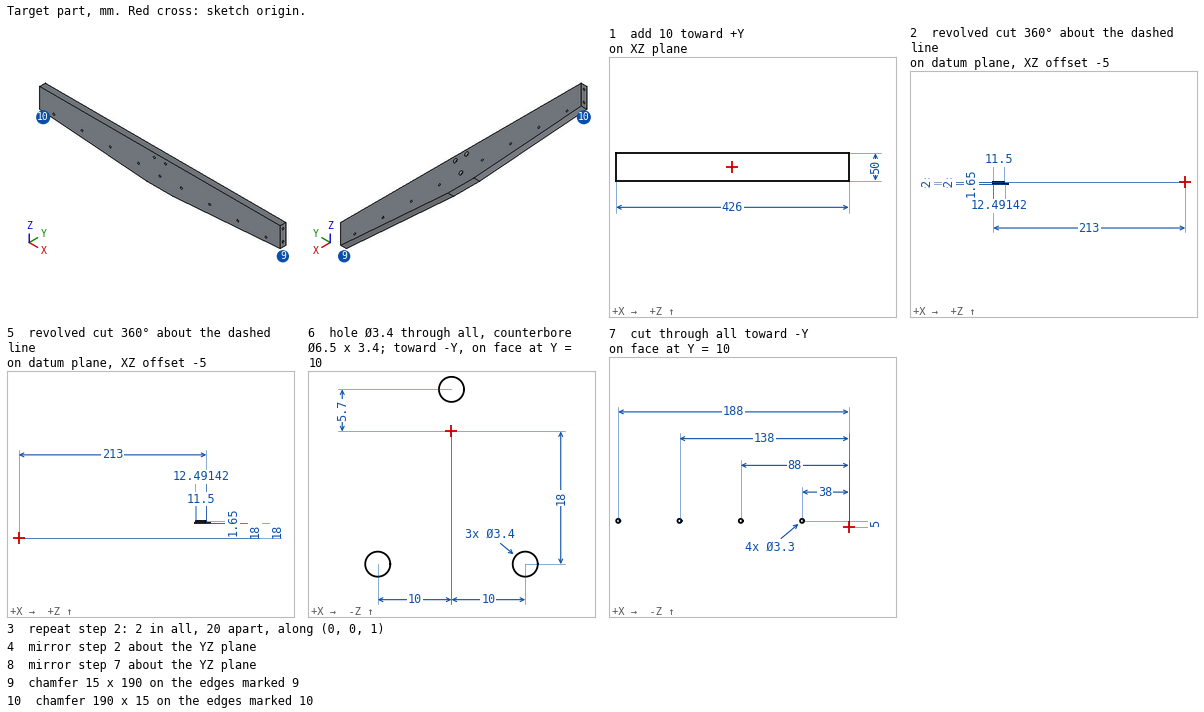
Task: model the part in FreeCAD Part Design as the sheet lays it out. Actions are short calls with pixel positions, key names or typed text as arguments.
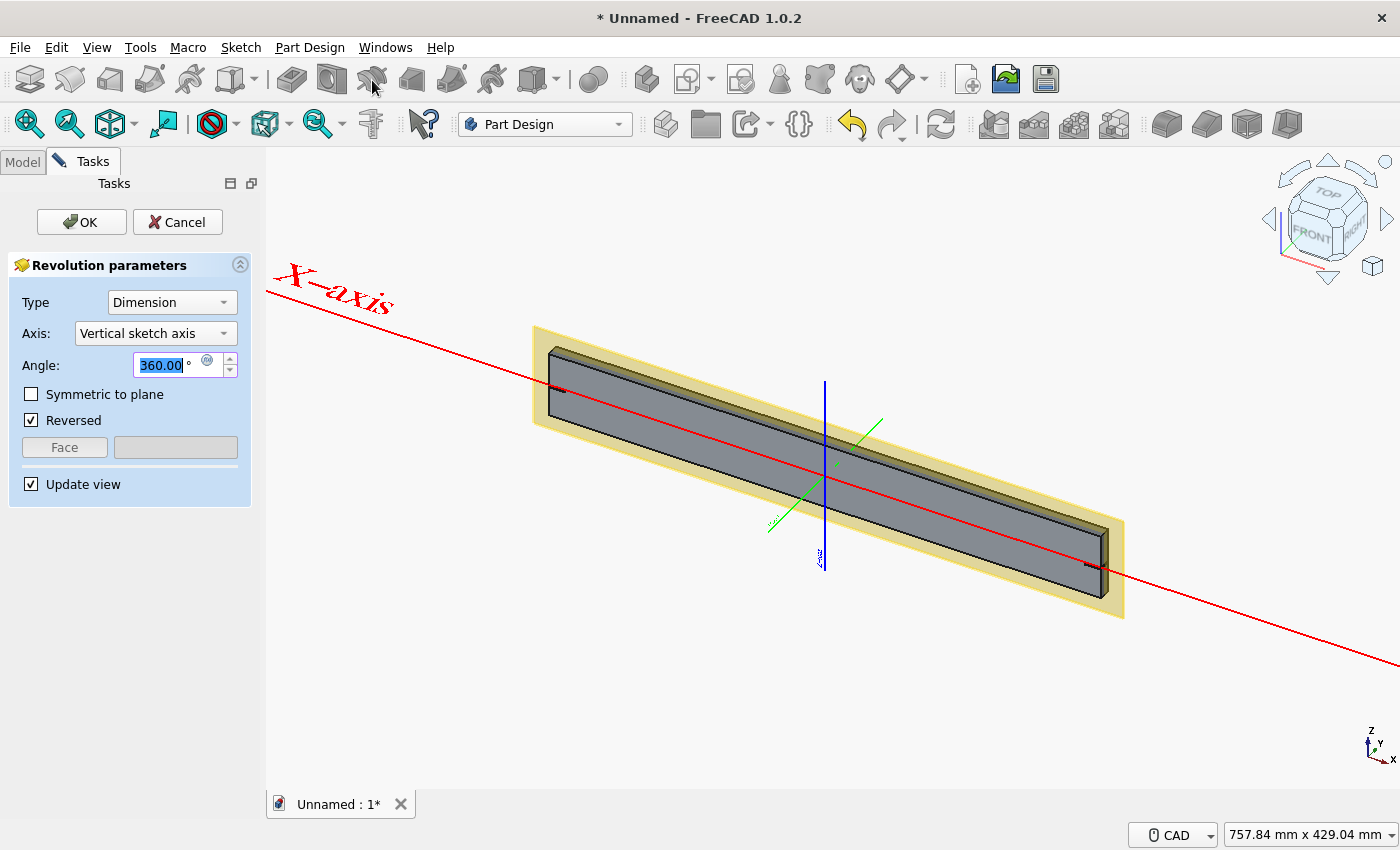
click(156, 334)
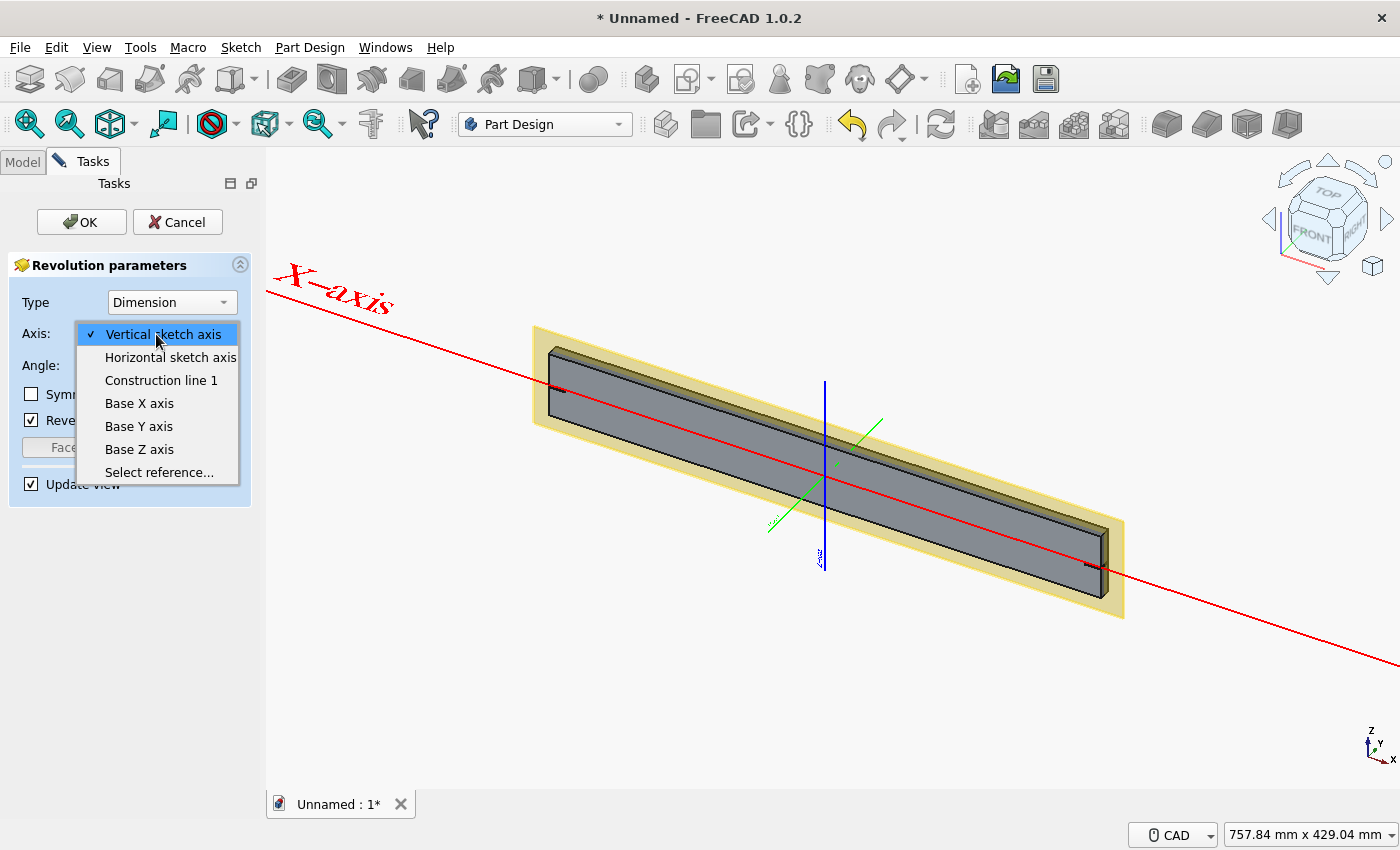
click(156, 380)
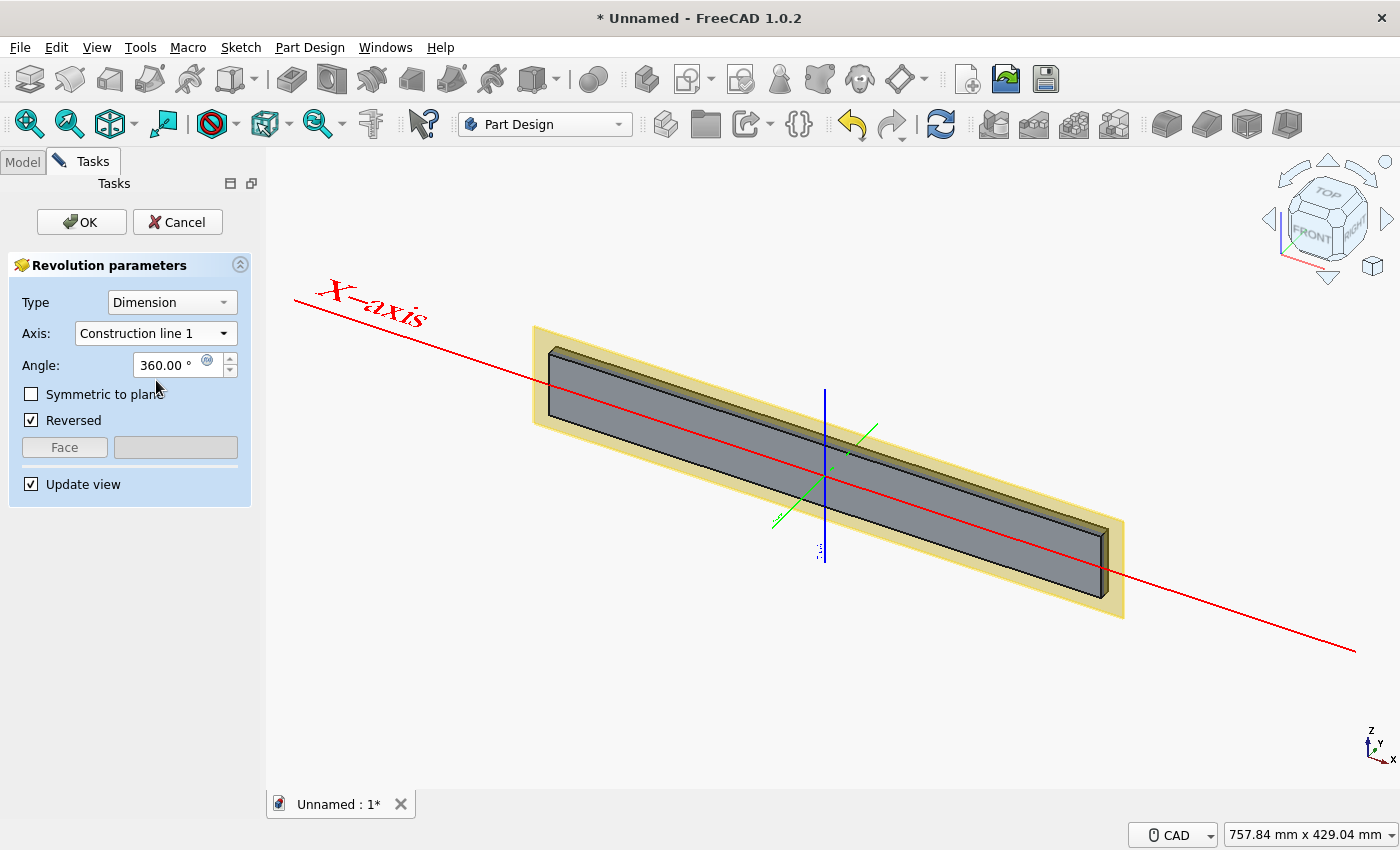
click(82, 222)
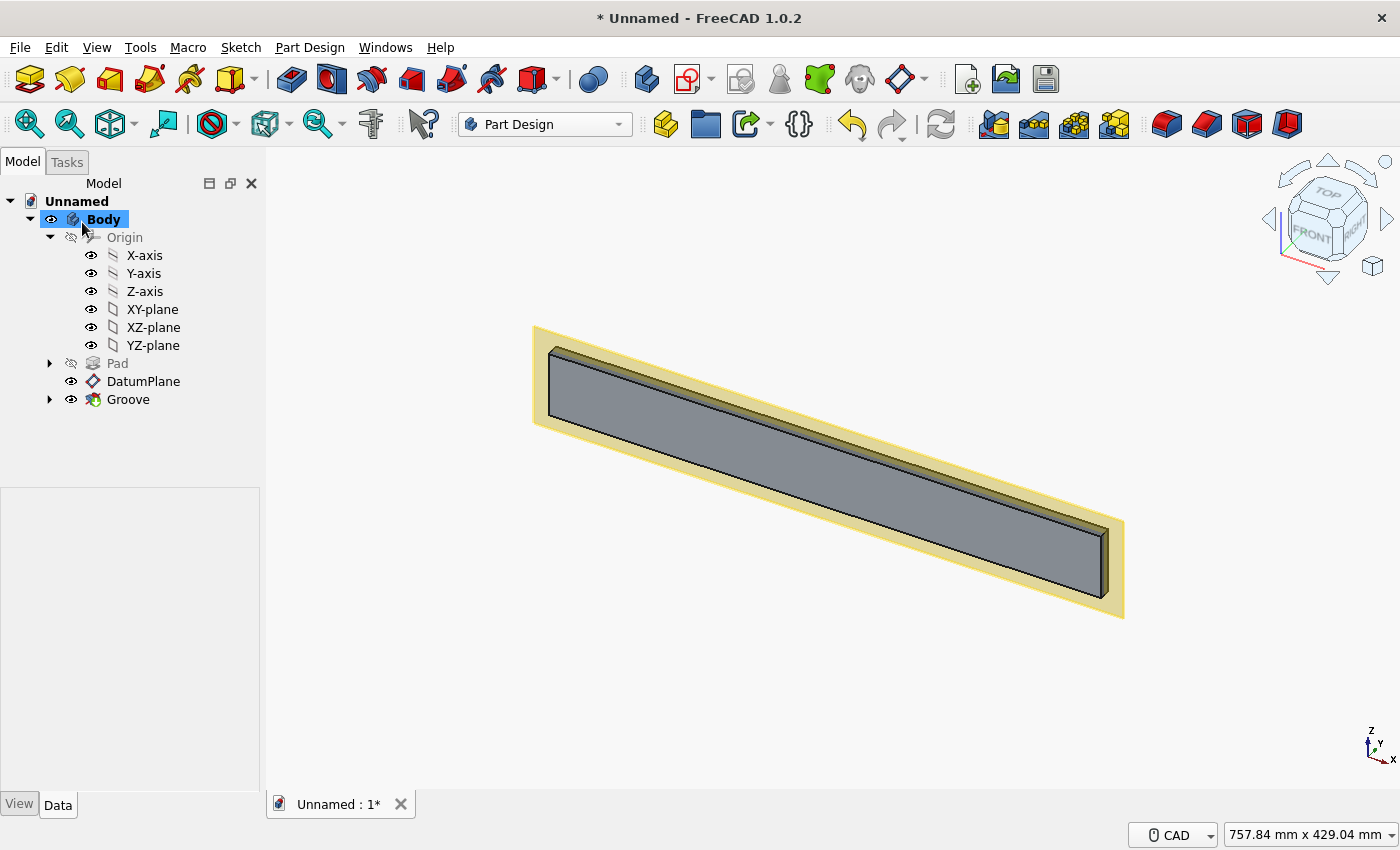
click(116, 381)
key(space)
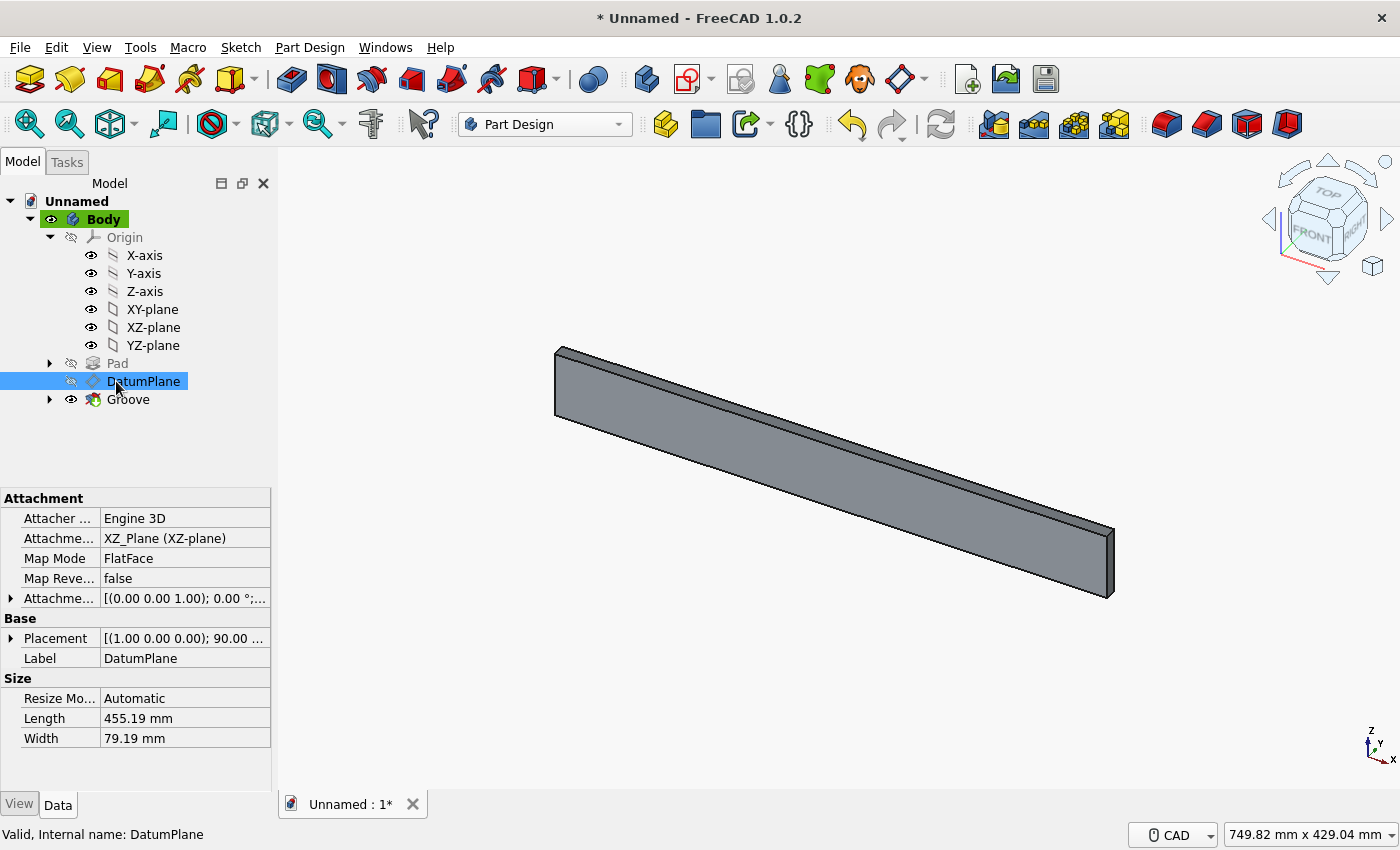
click(116, 399)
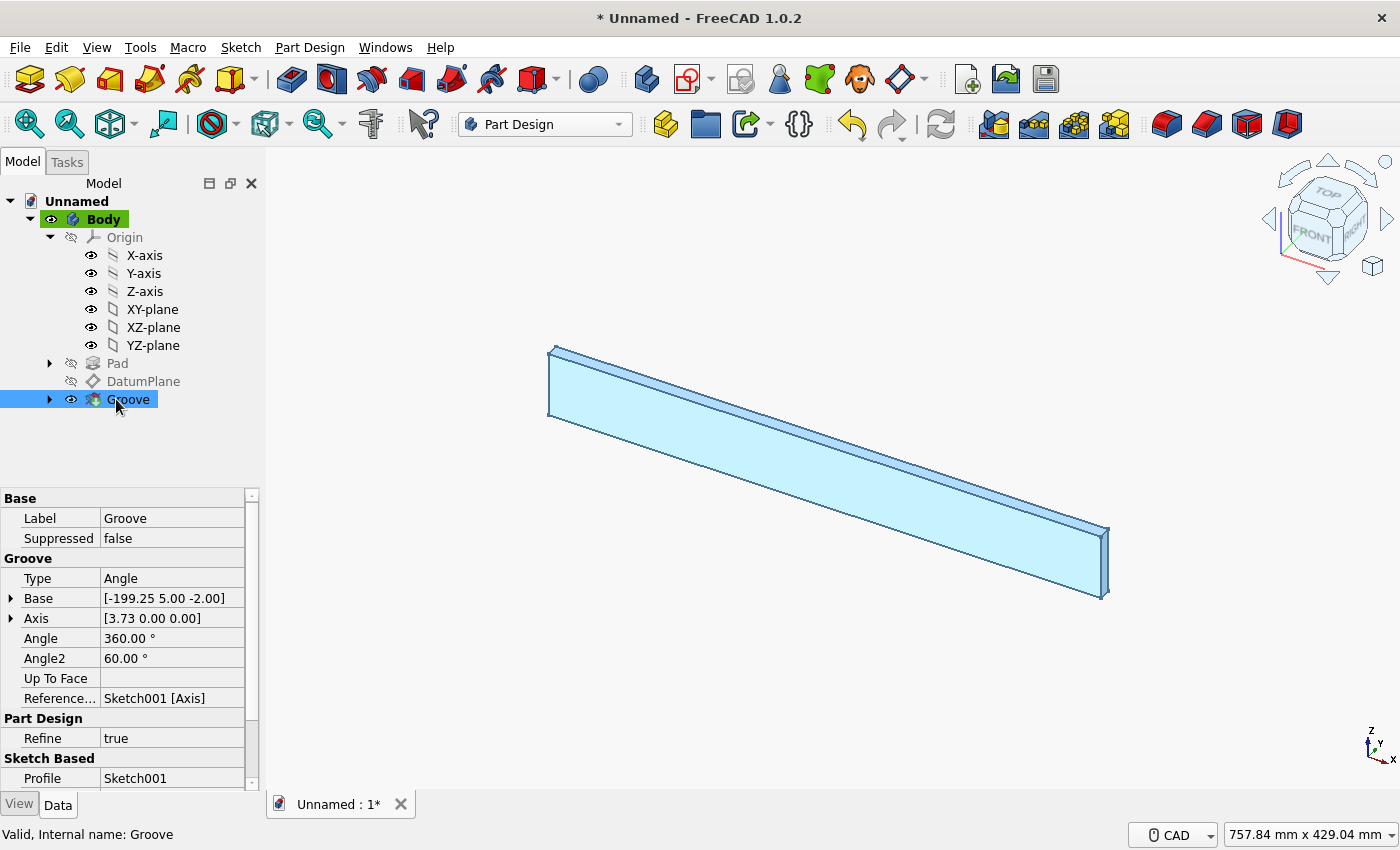
click(1034, 124)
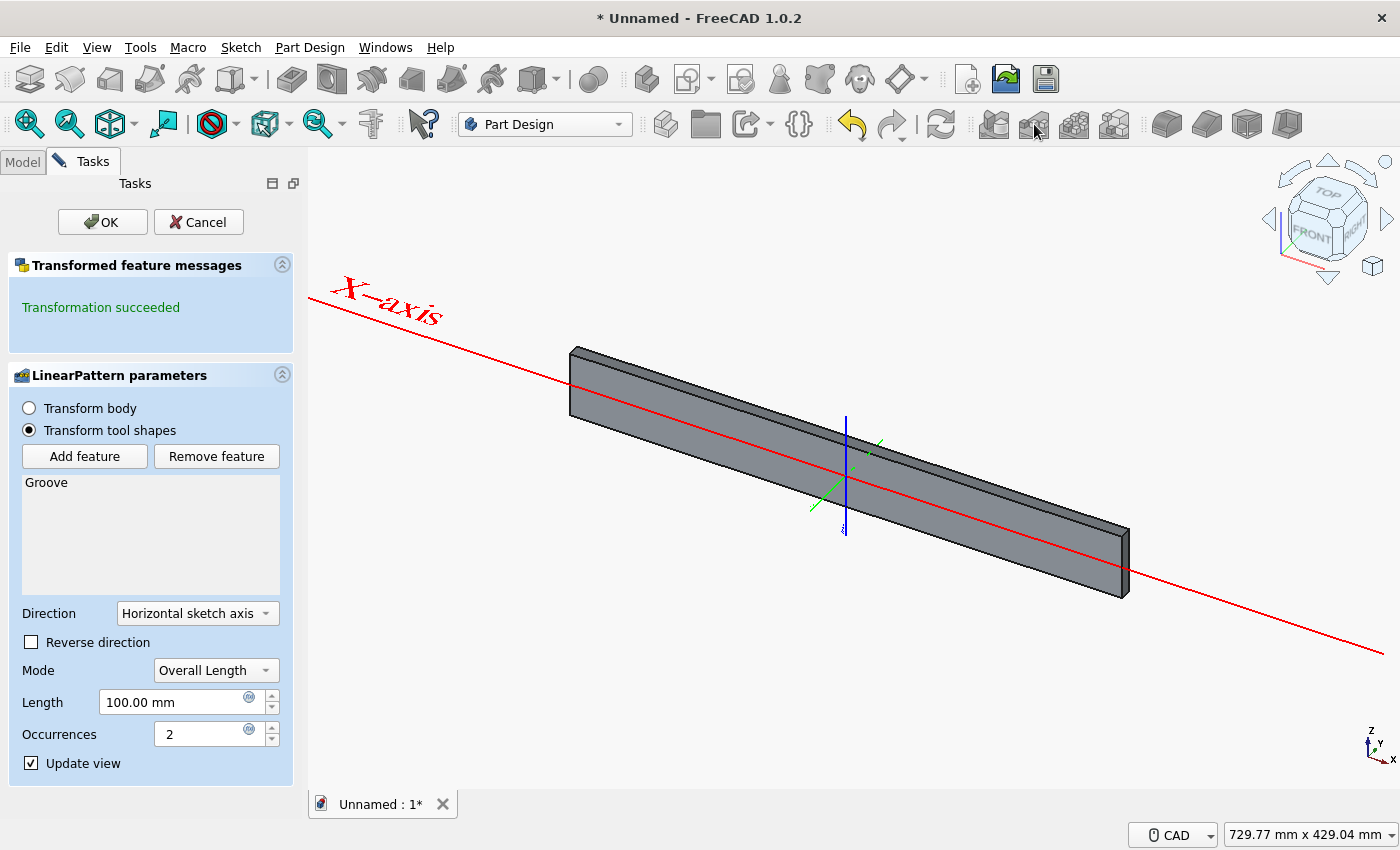
click(198, 614)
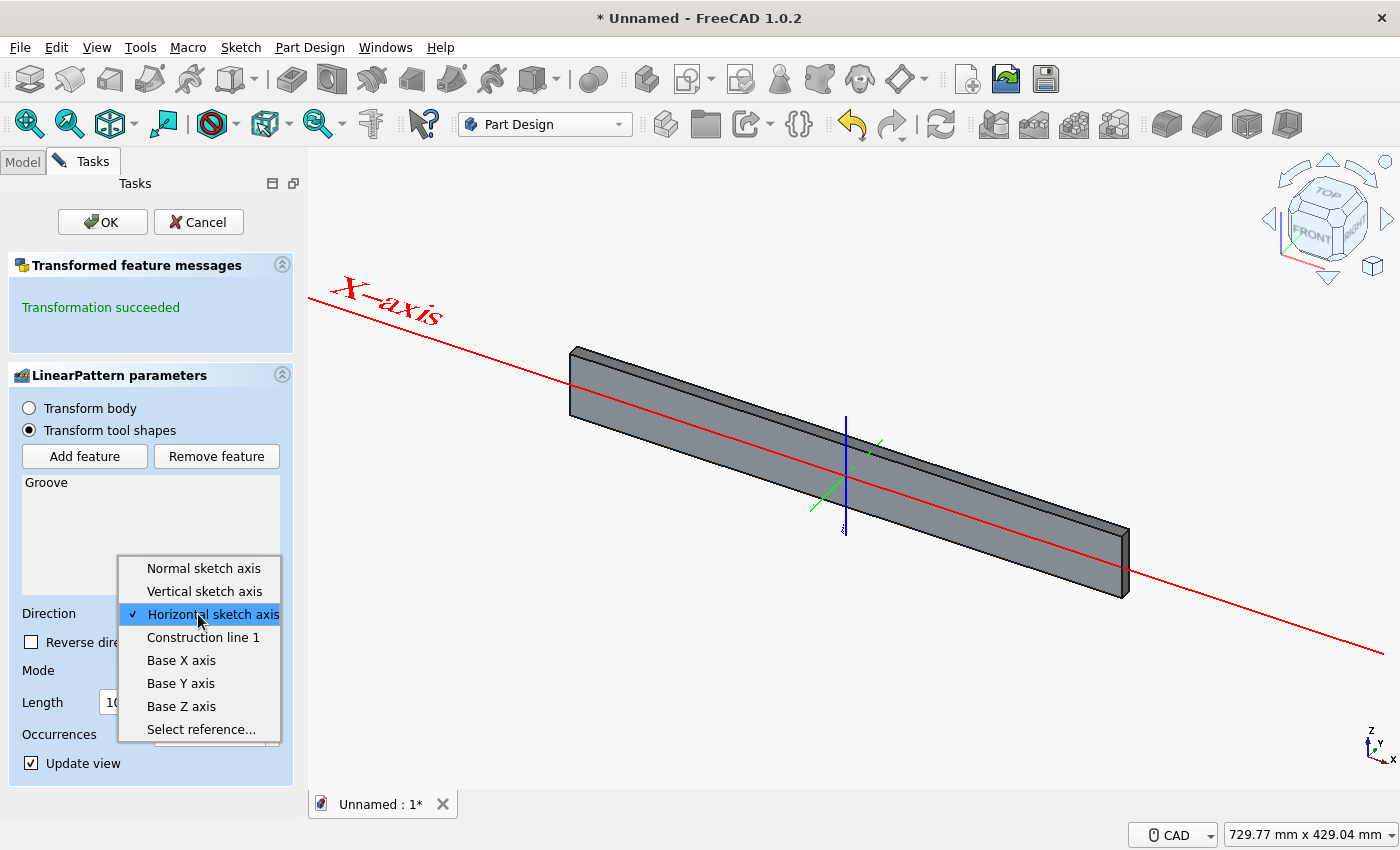
click(198, 706)